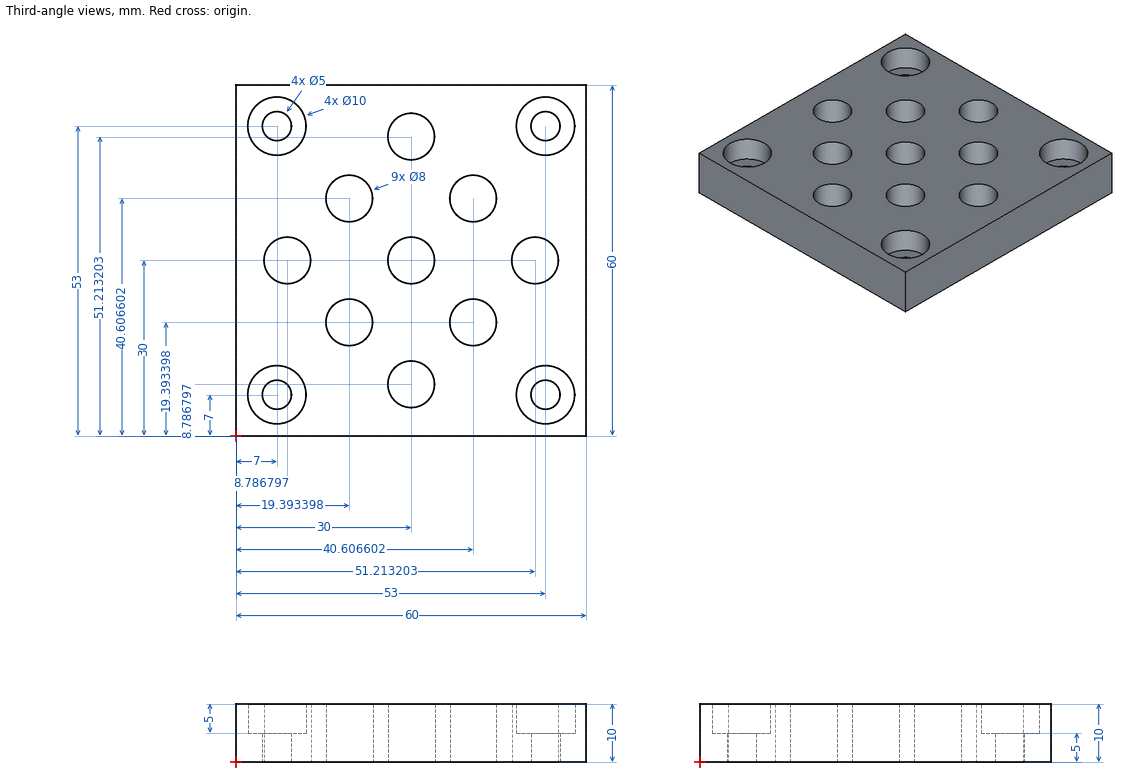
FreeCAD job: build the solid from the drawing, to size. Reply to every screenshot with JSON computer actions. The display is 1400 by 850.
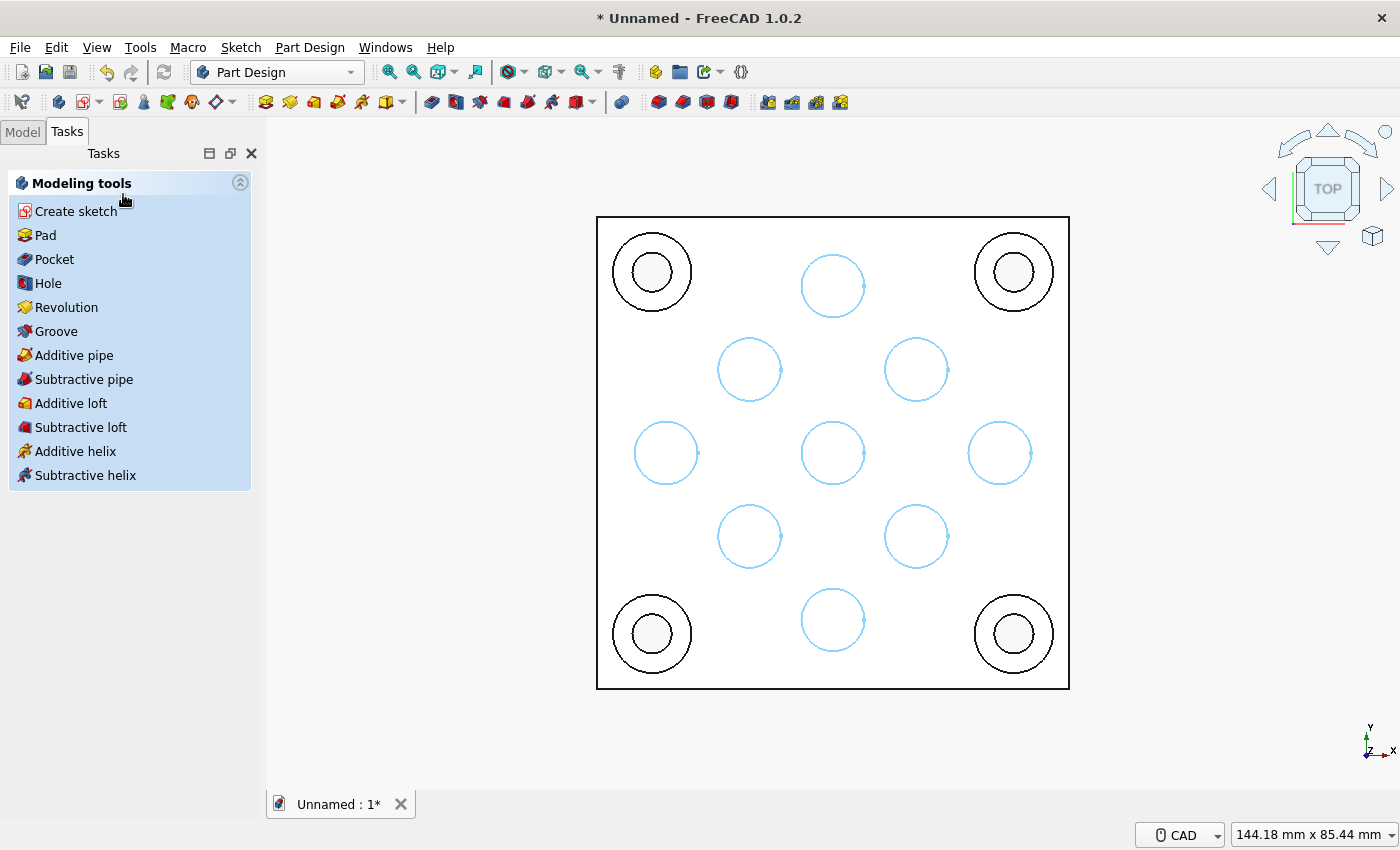
{"action": "left_click", "coordinate": [432, 102]}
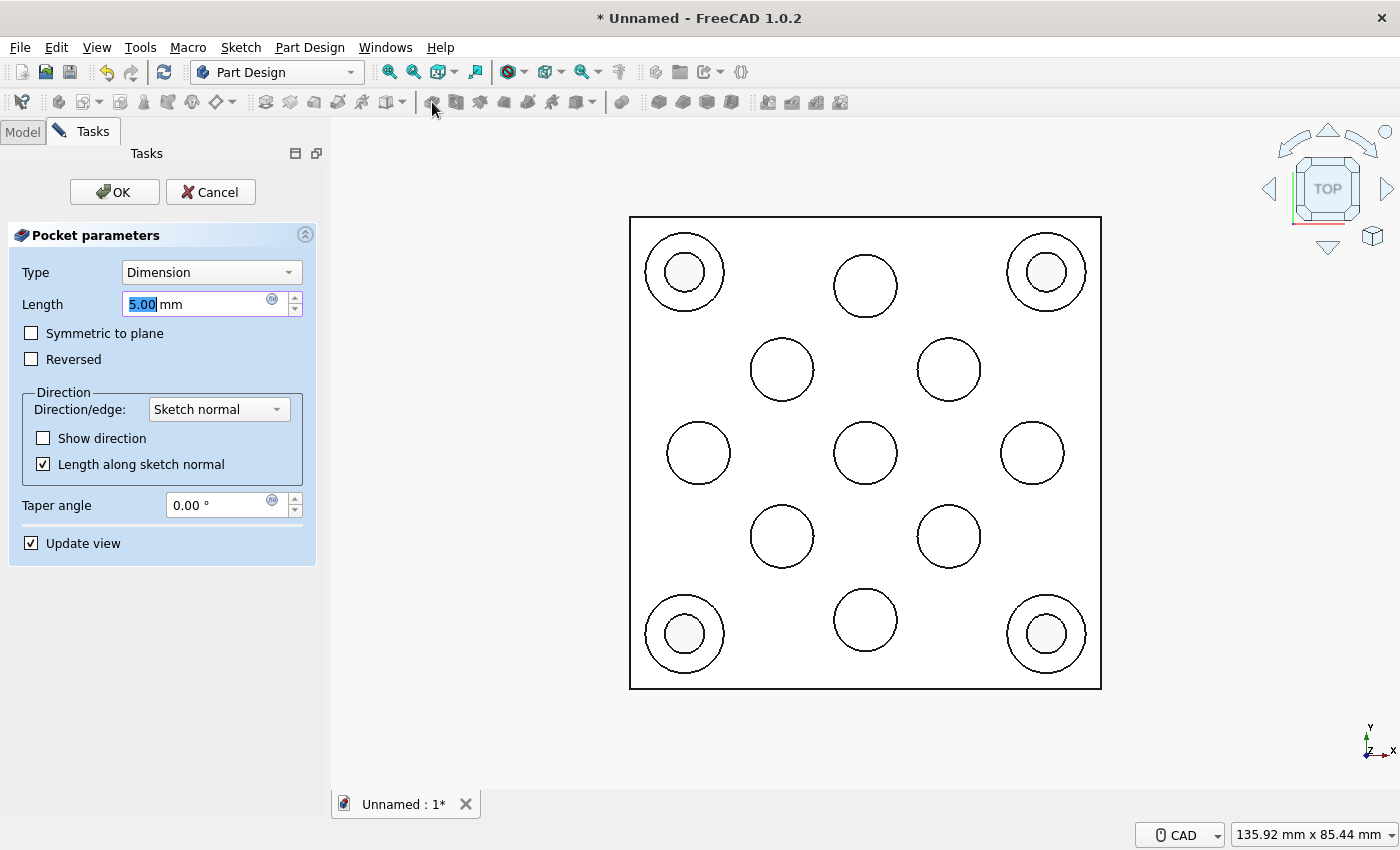
{"action": "type", "text": "10"}
{"action": "key", "text": "Tab"}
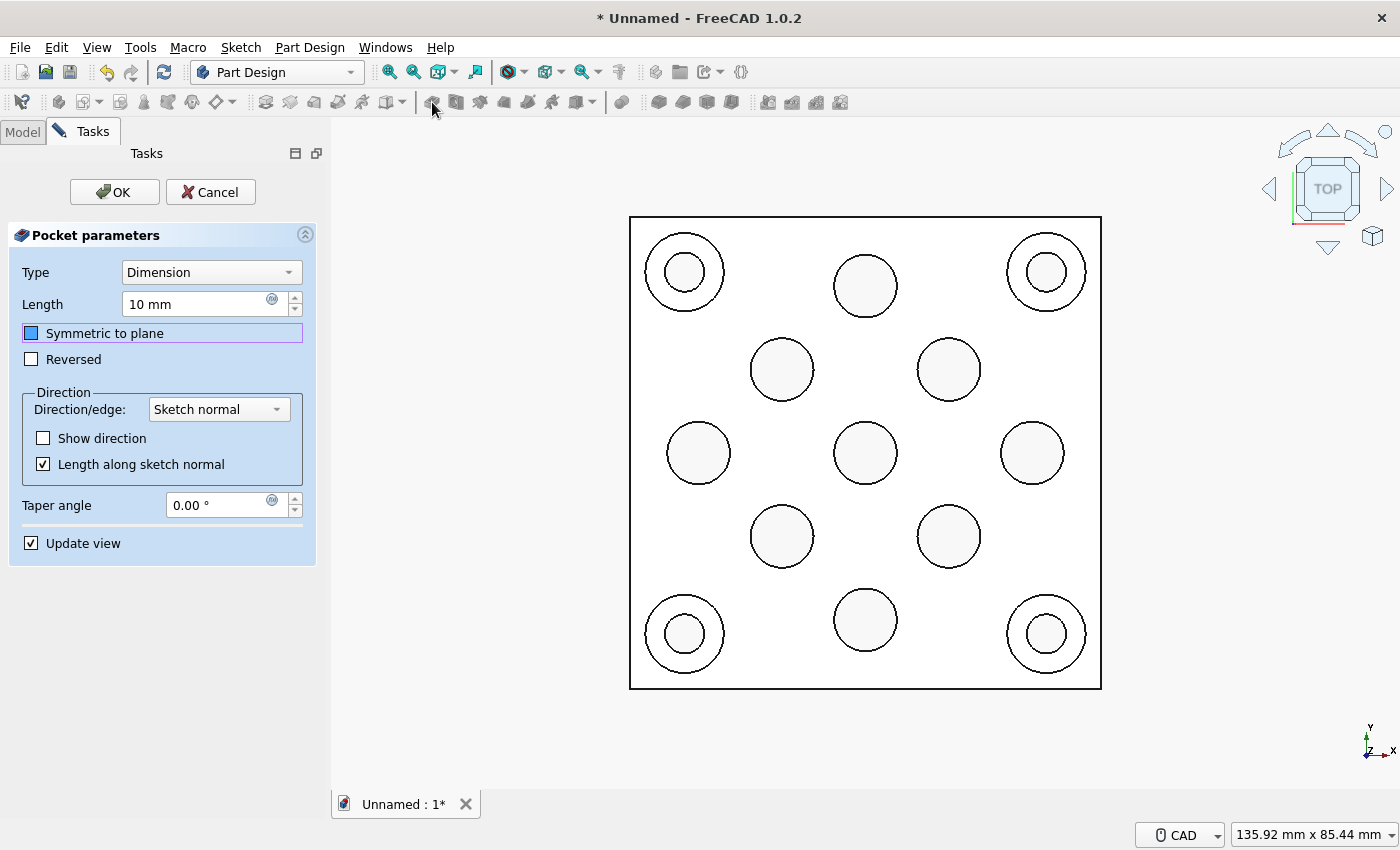
{"action": "left_click", "coordinate": [115, 192]}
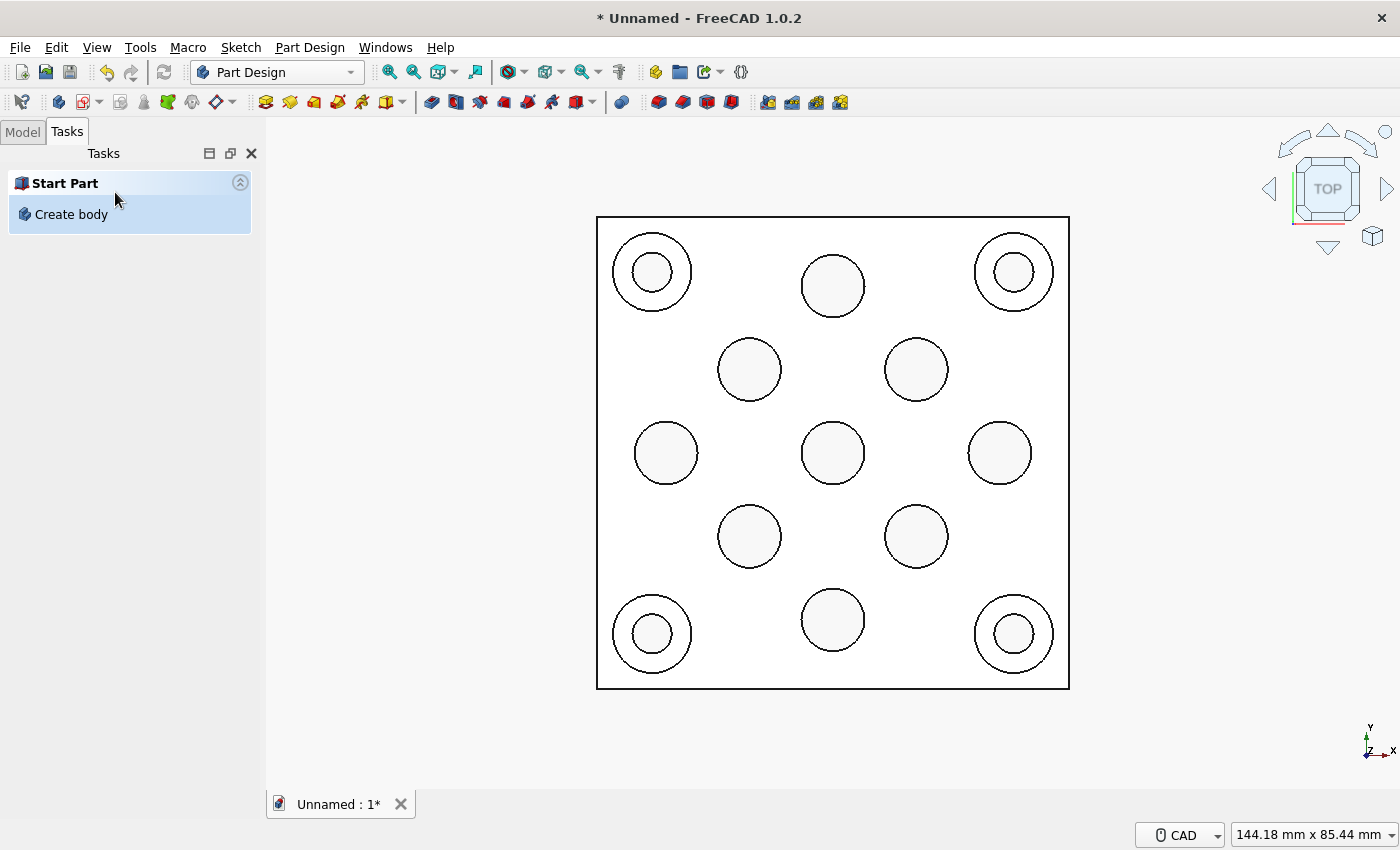
{"action": "key", "text": "0"}